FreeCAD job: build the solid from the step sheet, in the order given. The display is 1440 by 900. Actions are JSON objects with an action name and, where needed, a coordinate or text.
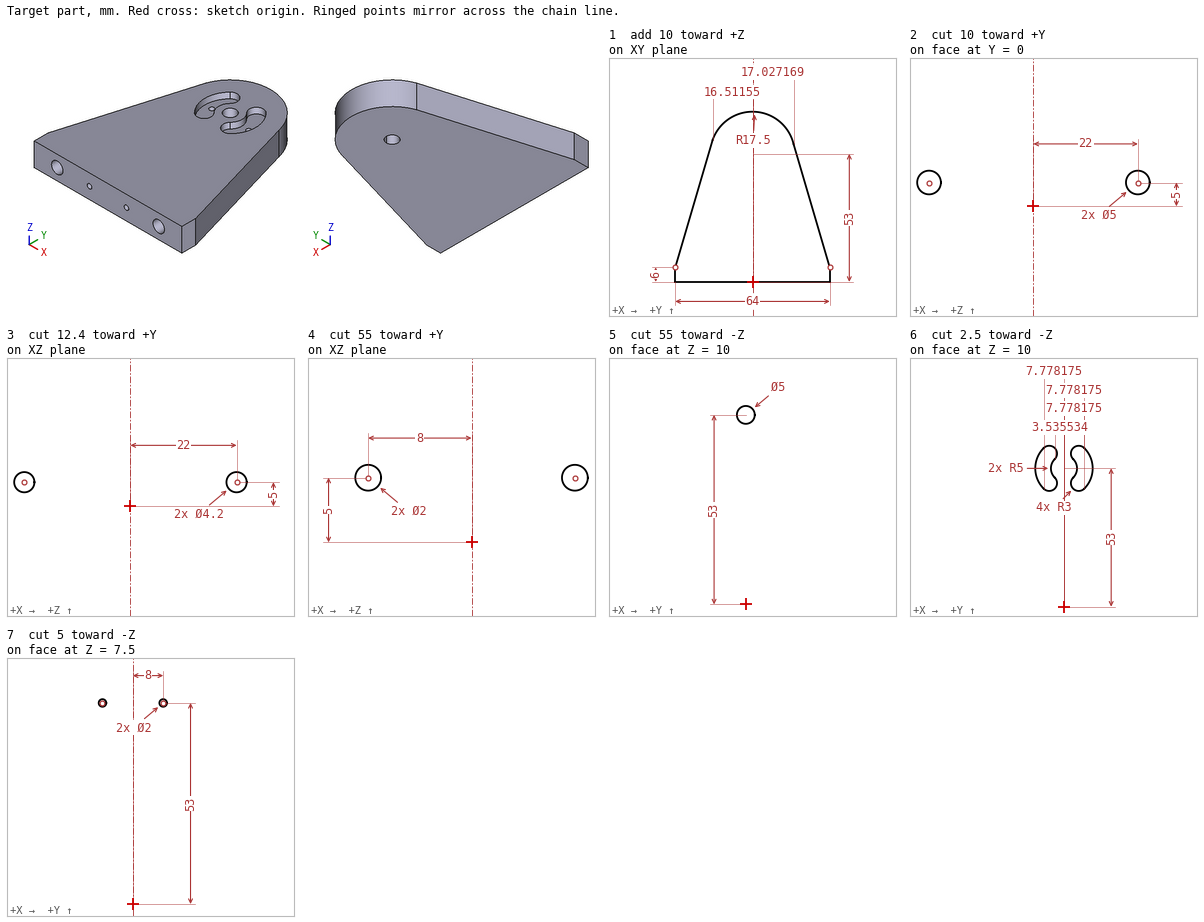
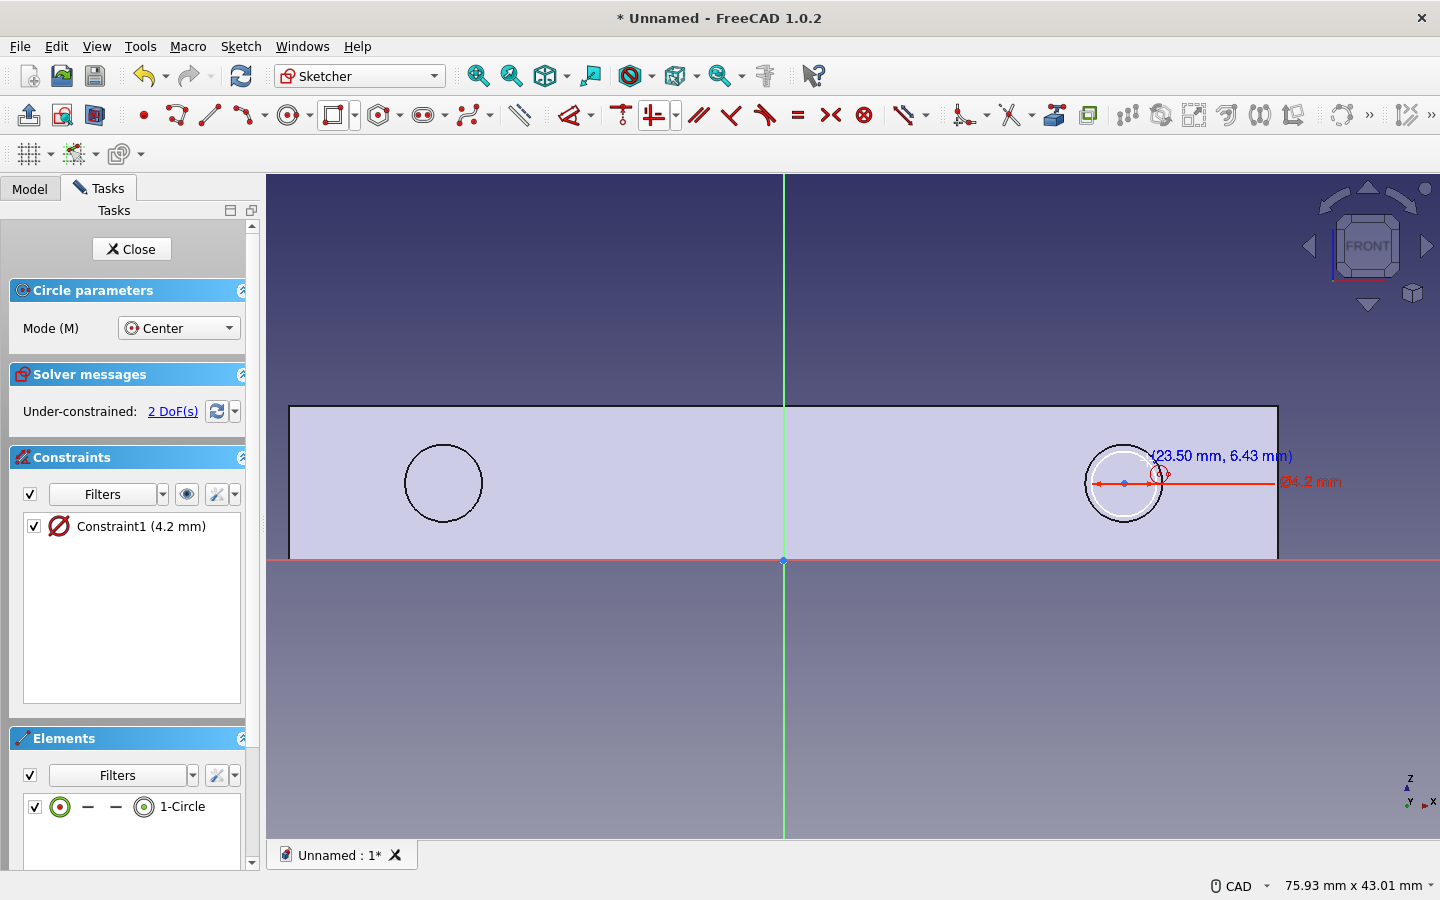
{"action": "left_click", "coordinate": [444, 483]}
{"action": "mouse_move", "coordinate": [467, 460]}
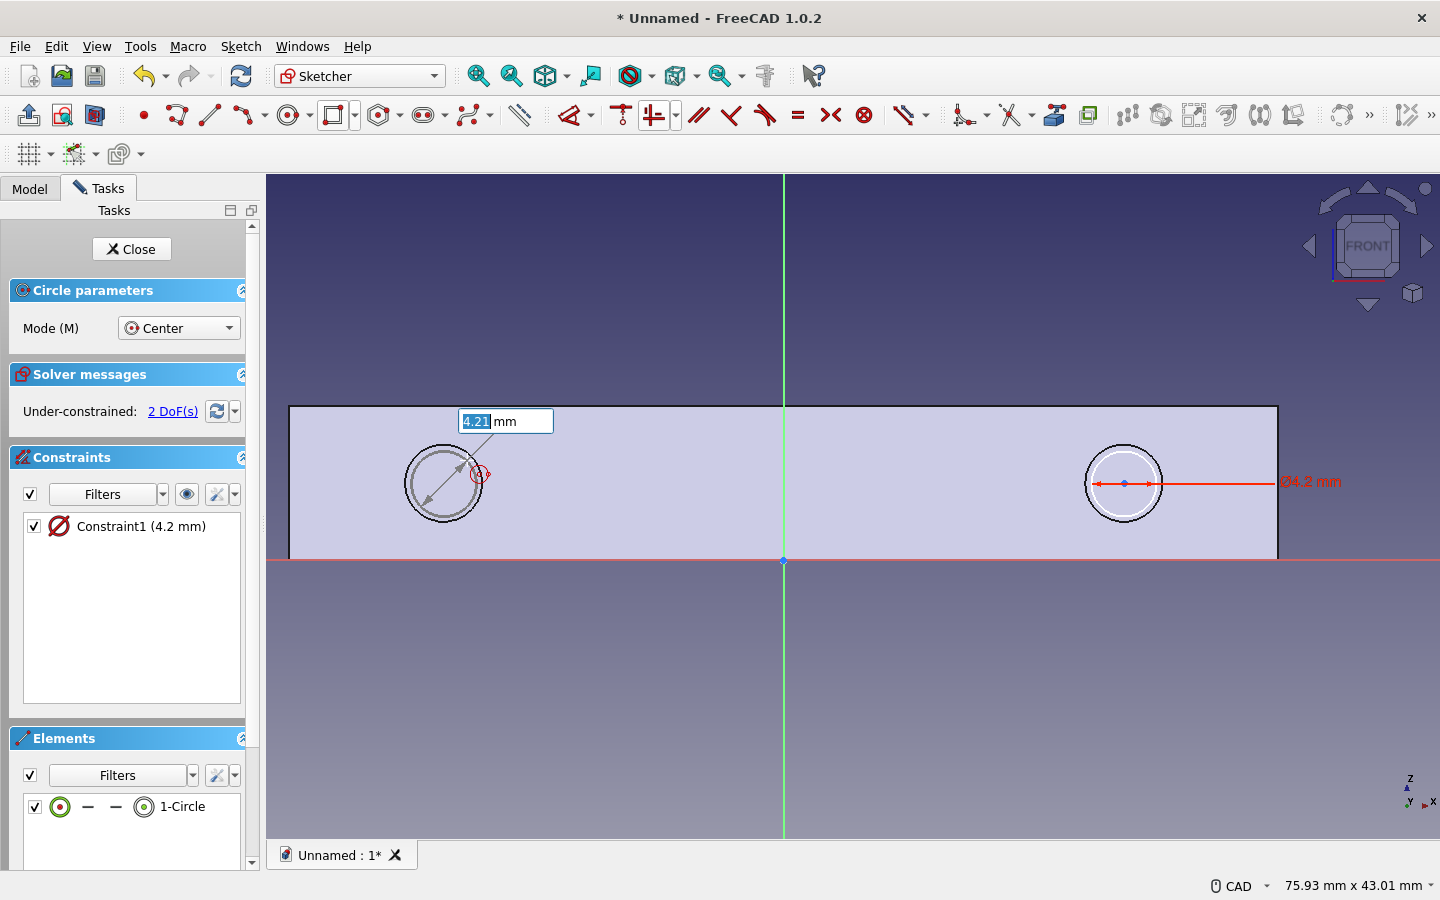
{"action": "type", "text": "4.2"}
{"action": "key", "text": "Return"}
{"action": "key", "text": "Escape"}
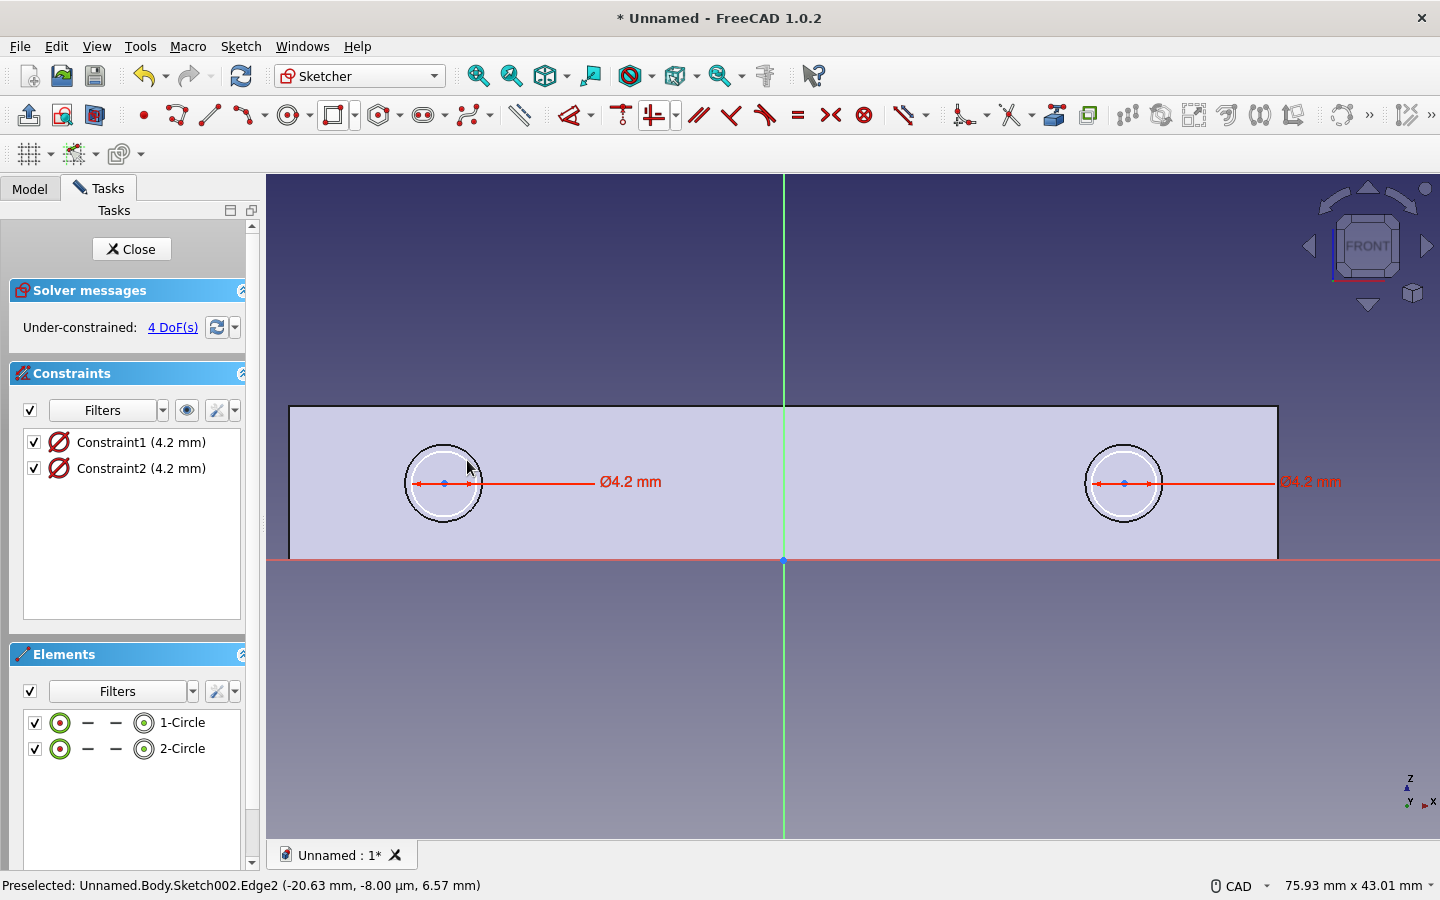
{"action": "left_click", "coordinate": [1124, 484]}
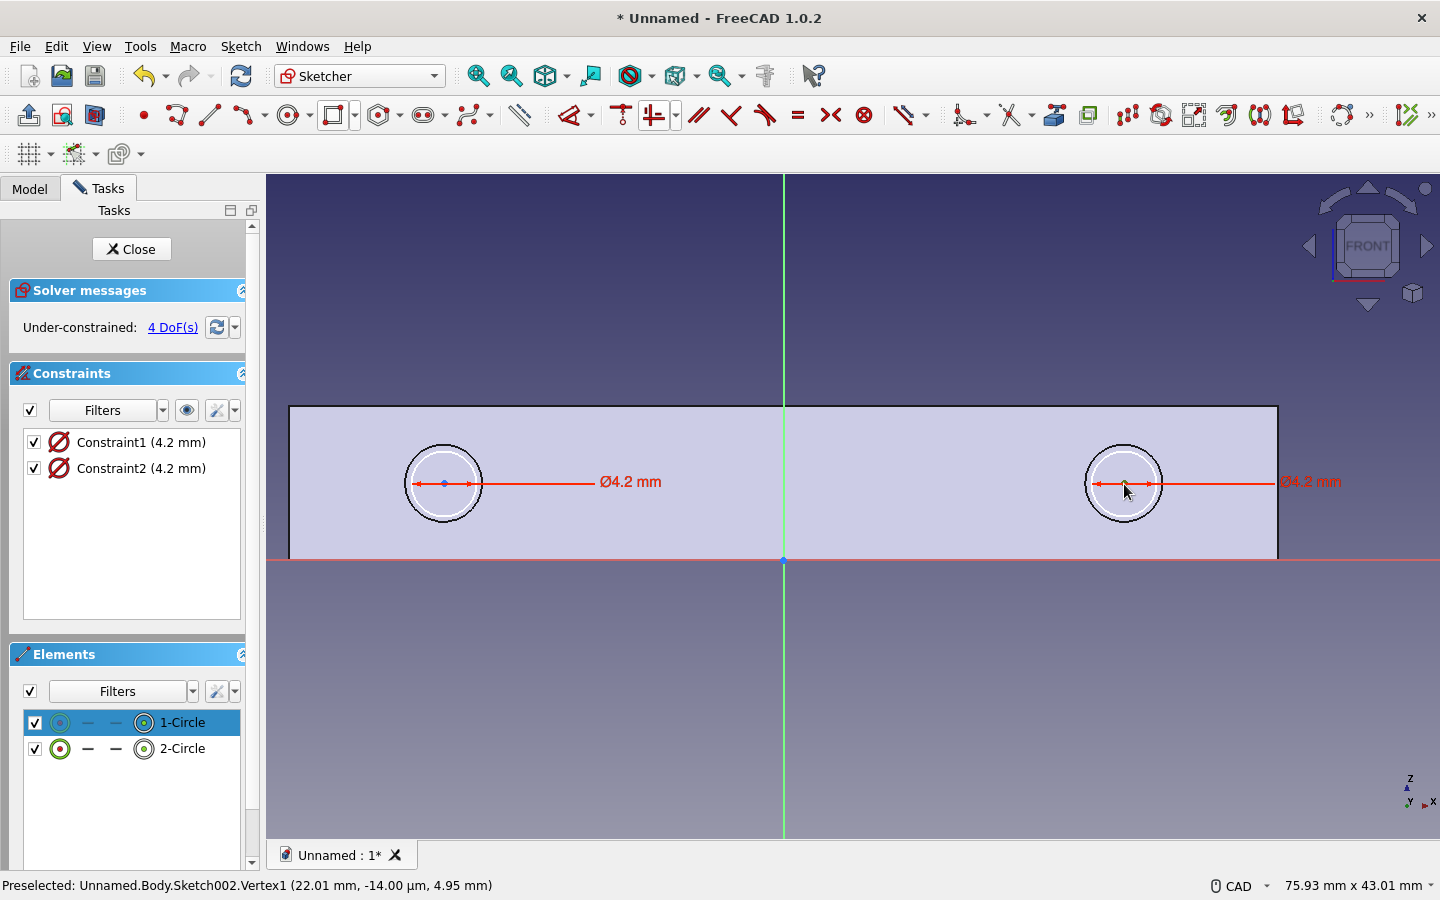
{"action": "left_click", "coordinate": [444, 484]}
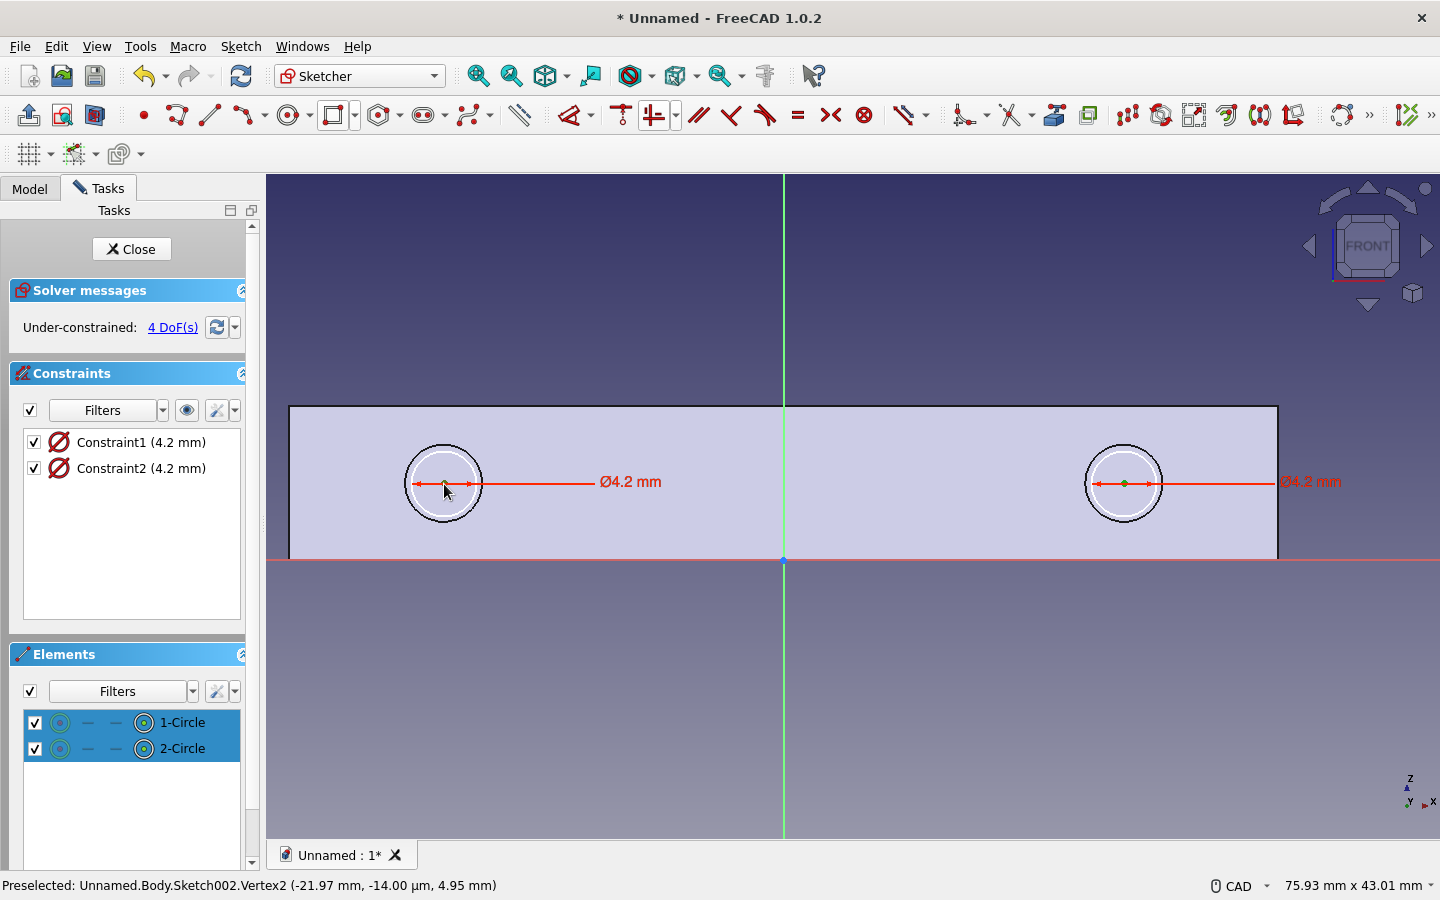
{"action": "left_click", "coordinate": [784, 768]}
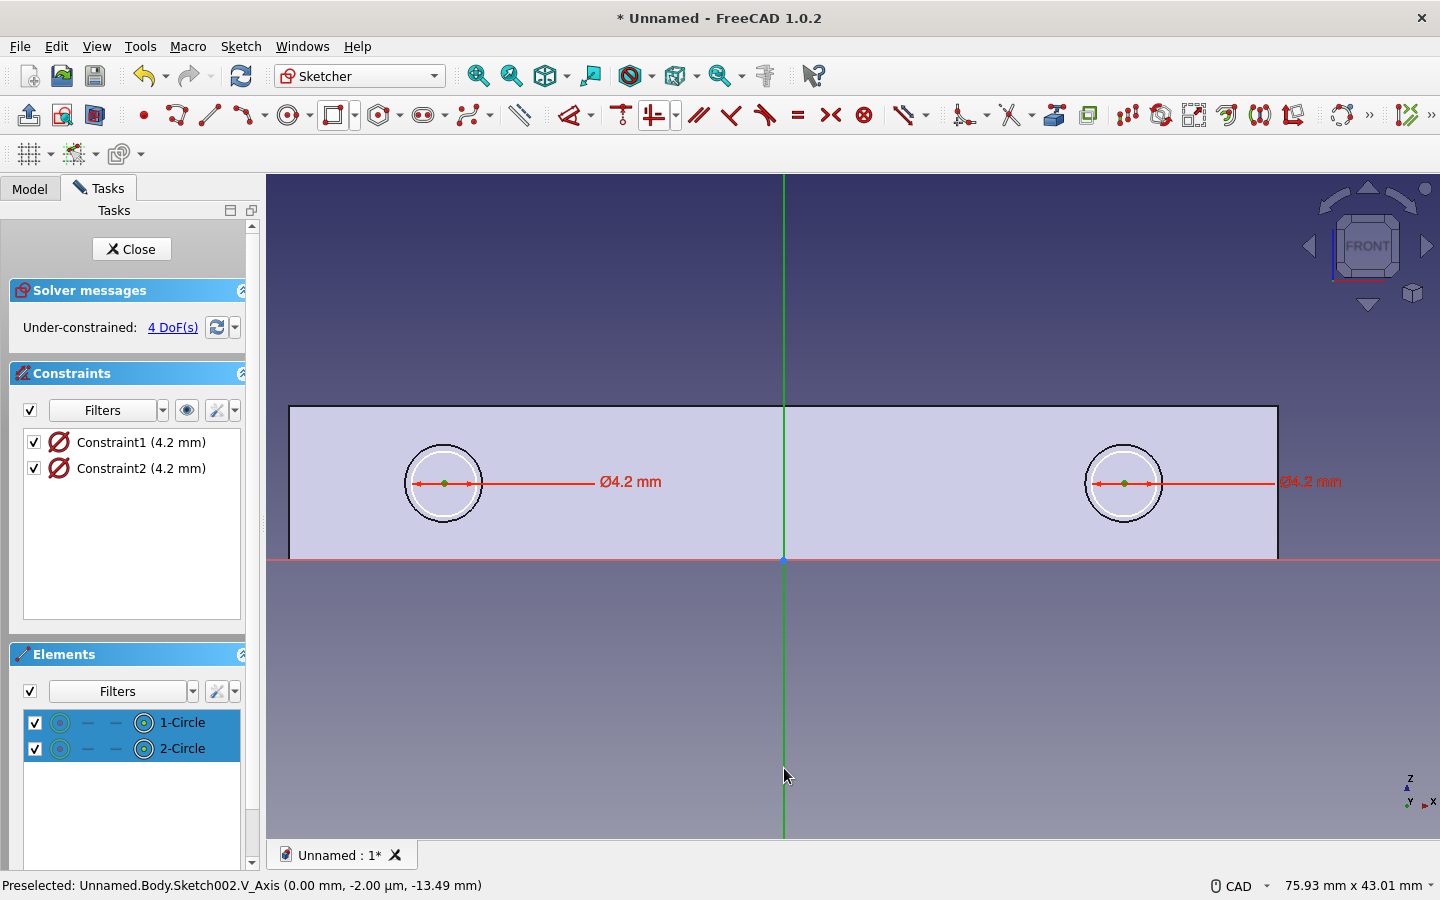
{"action": "left_click", "coordinate": [831, 116]}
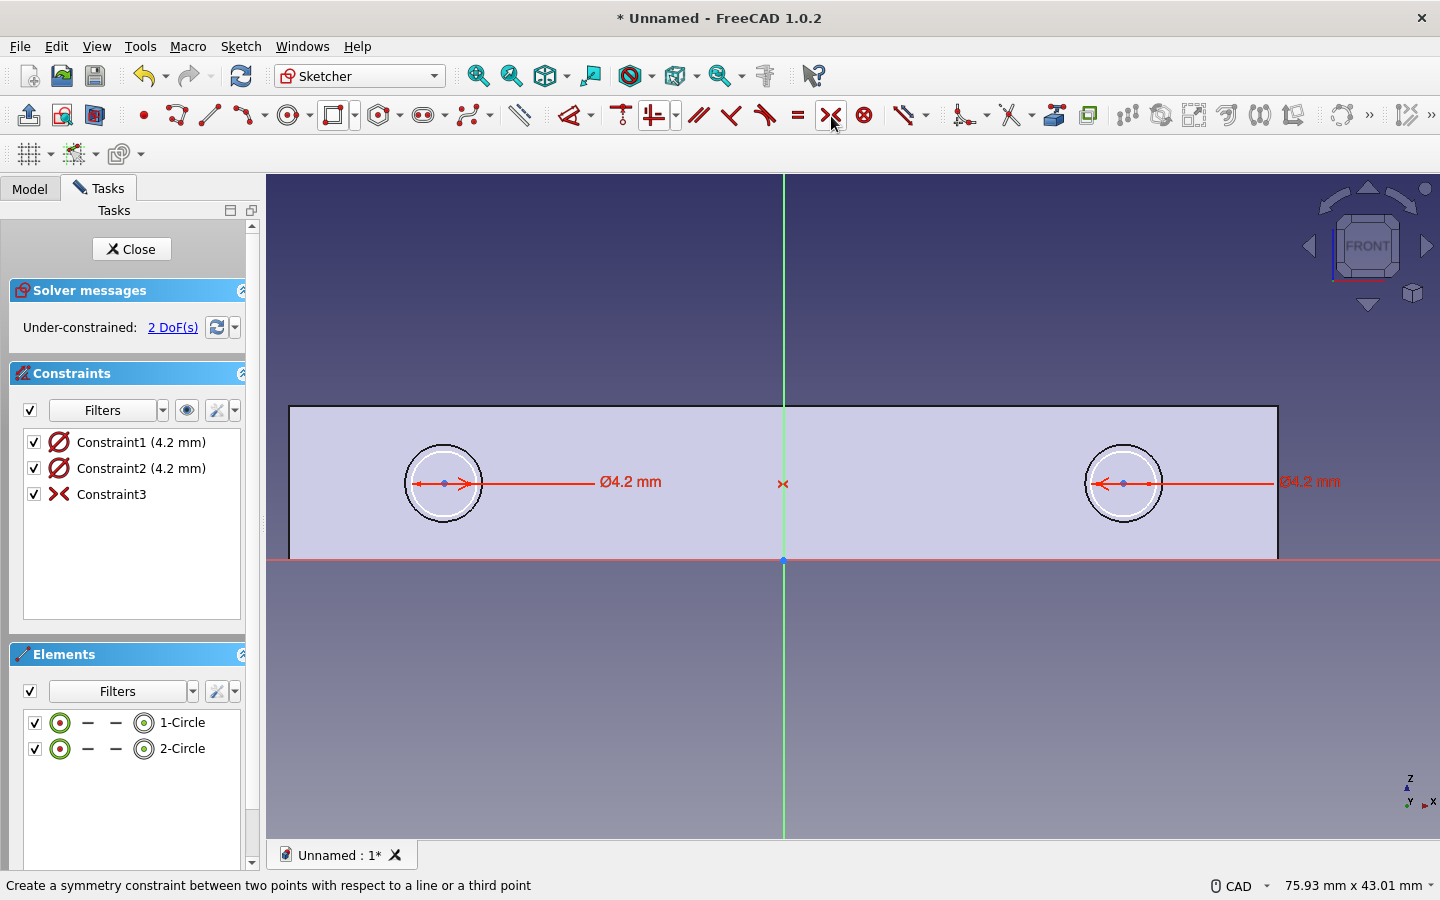
{"action": "key", "text": "d"}